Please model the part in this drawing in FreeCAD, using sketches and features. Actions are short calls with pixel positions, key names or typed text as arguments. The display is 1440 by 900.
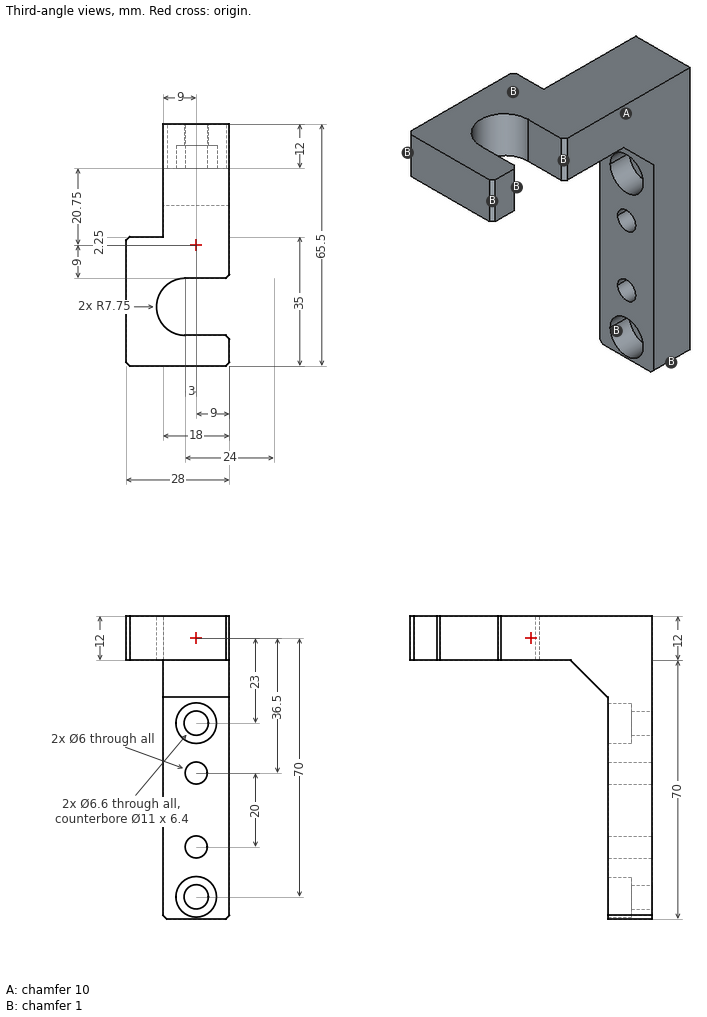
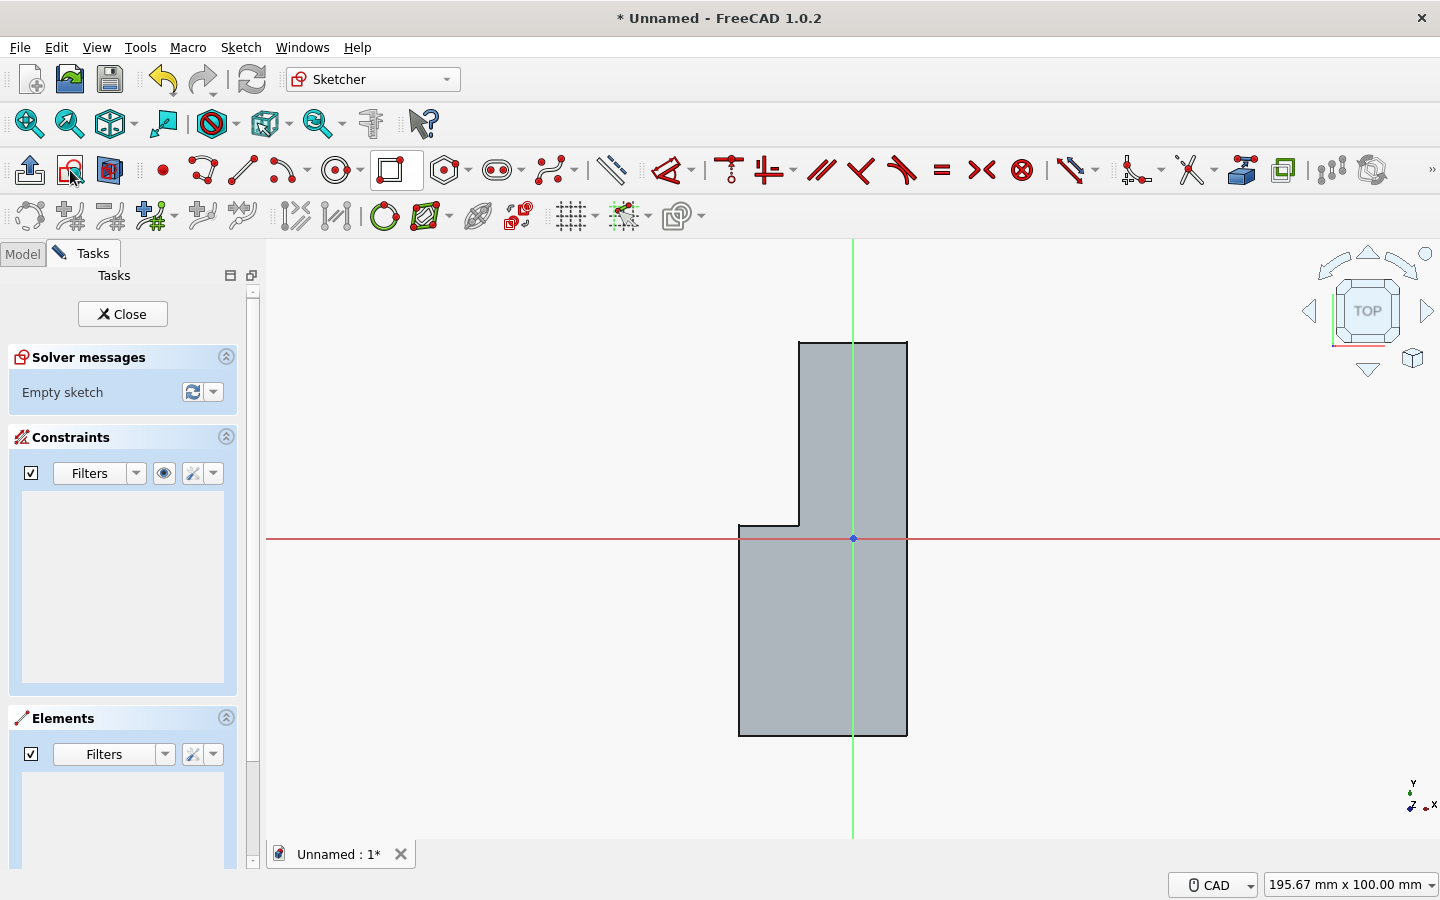
scroll(978, 655, up, 5)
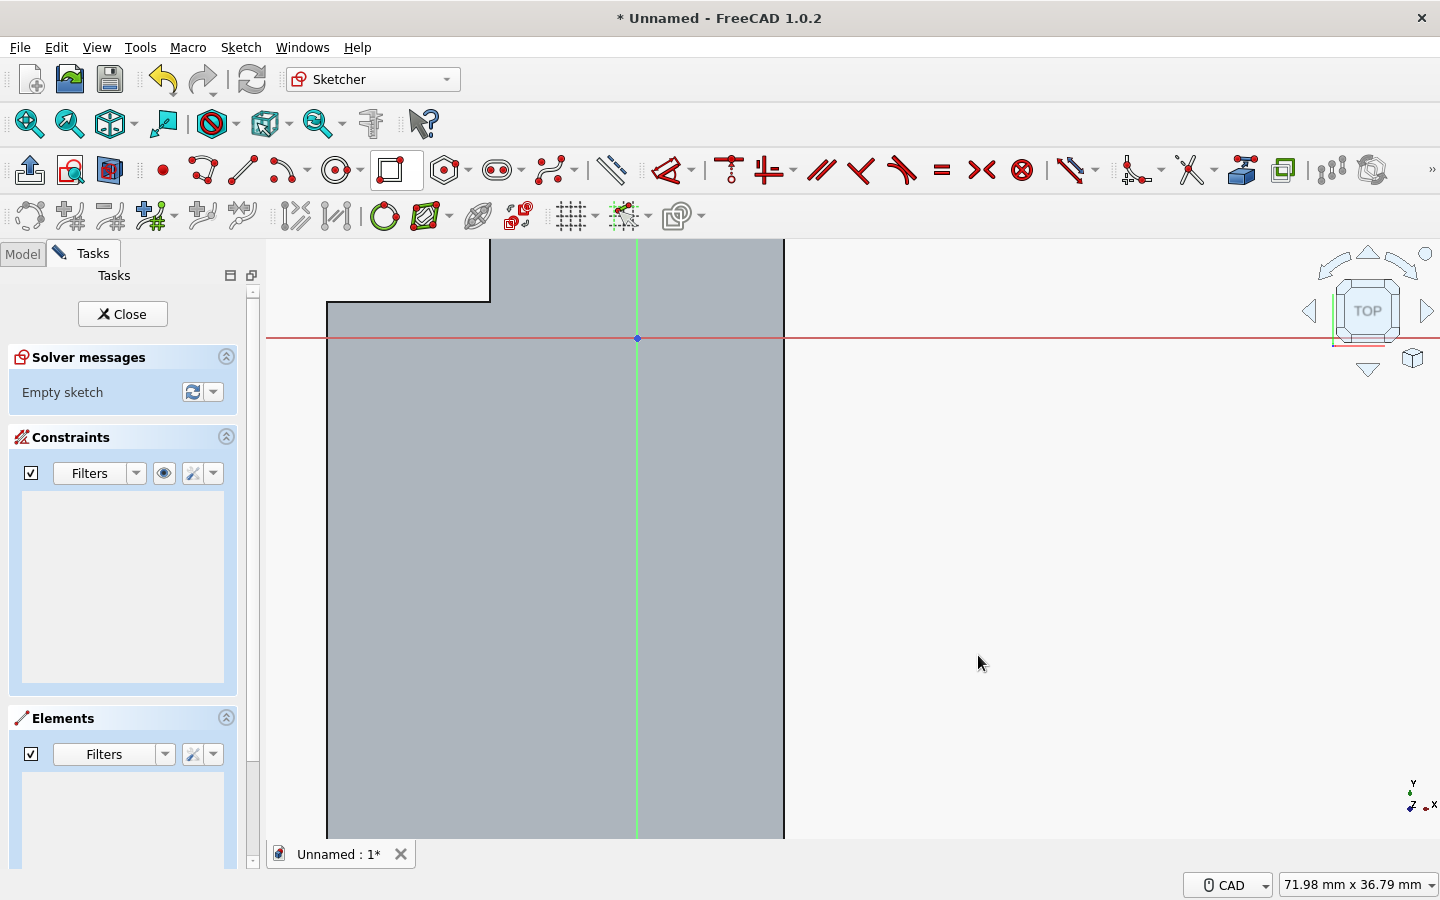
click(498, 170)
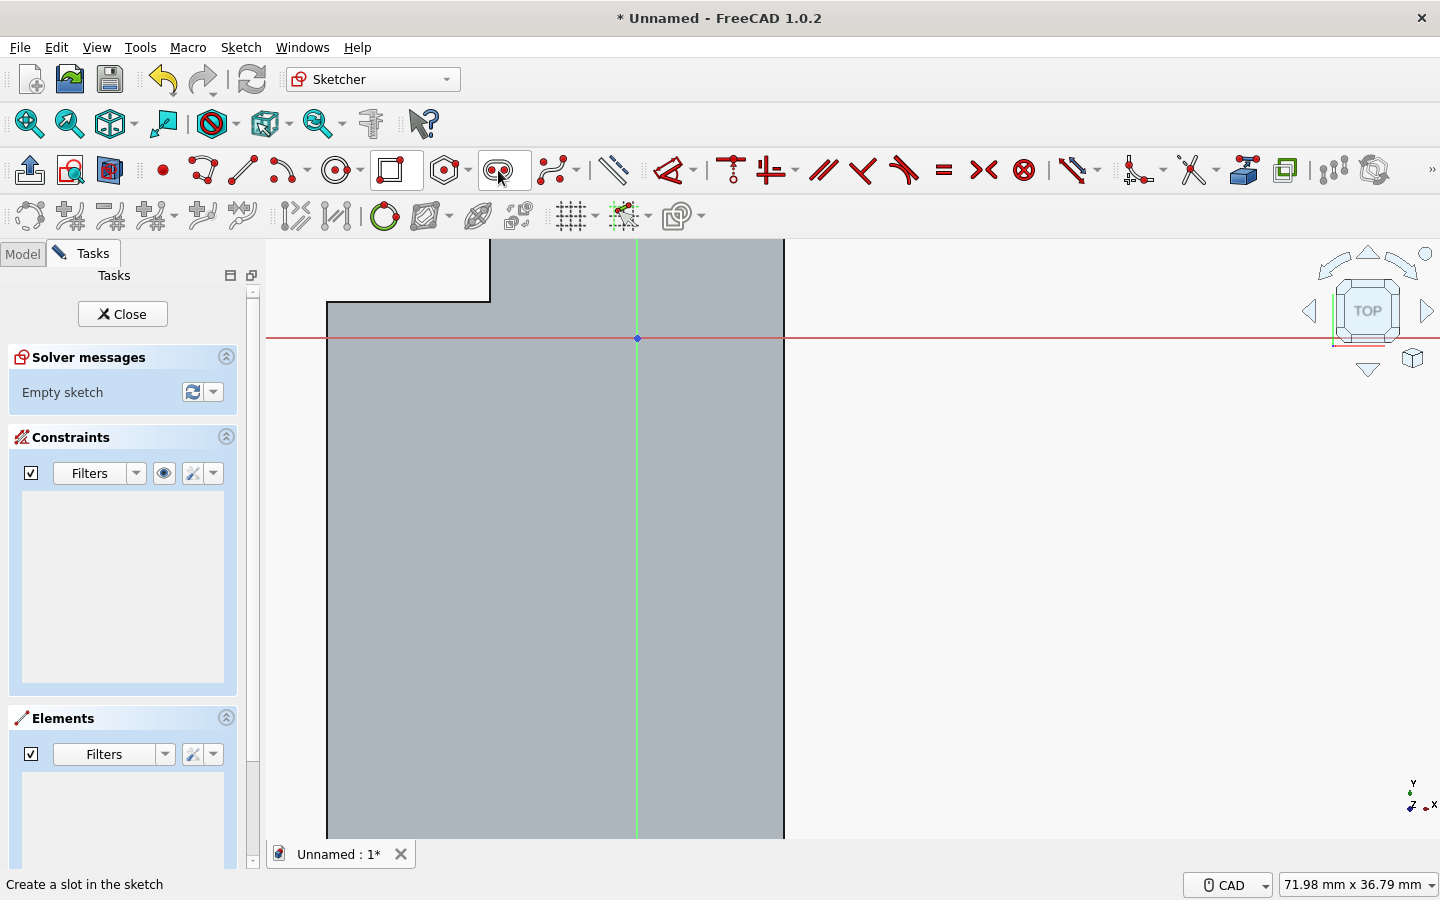
click(588, 612)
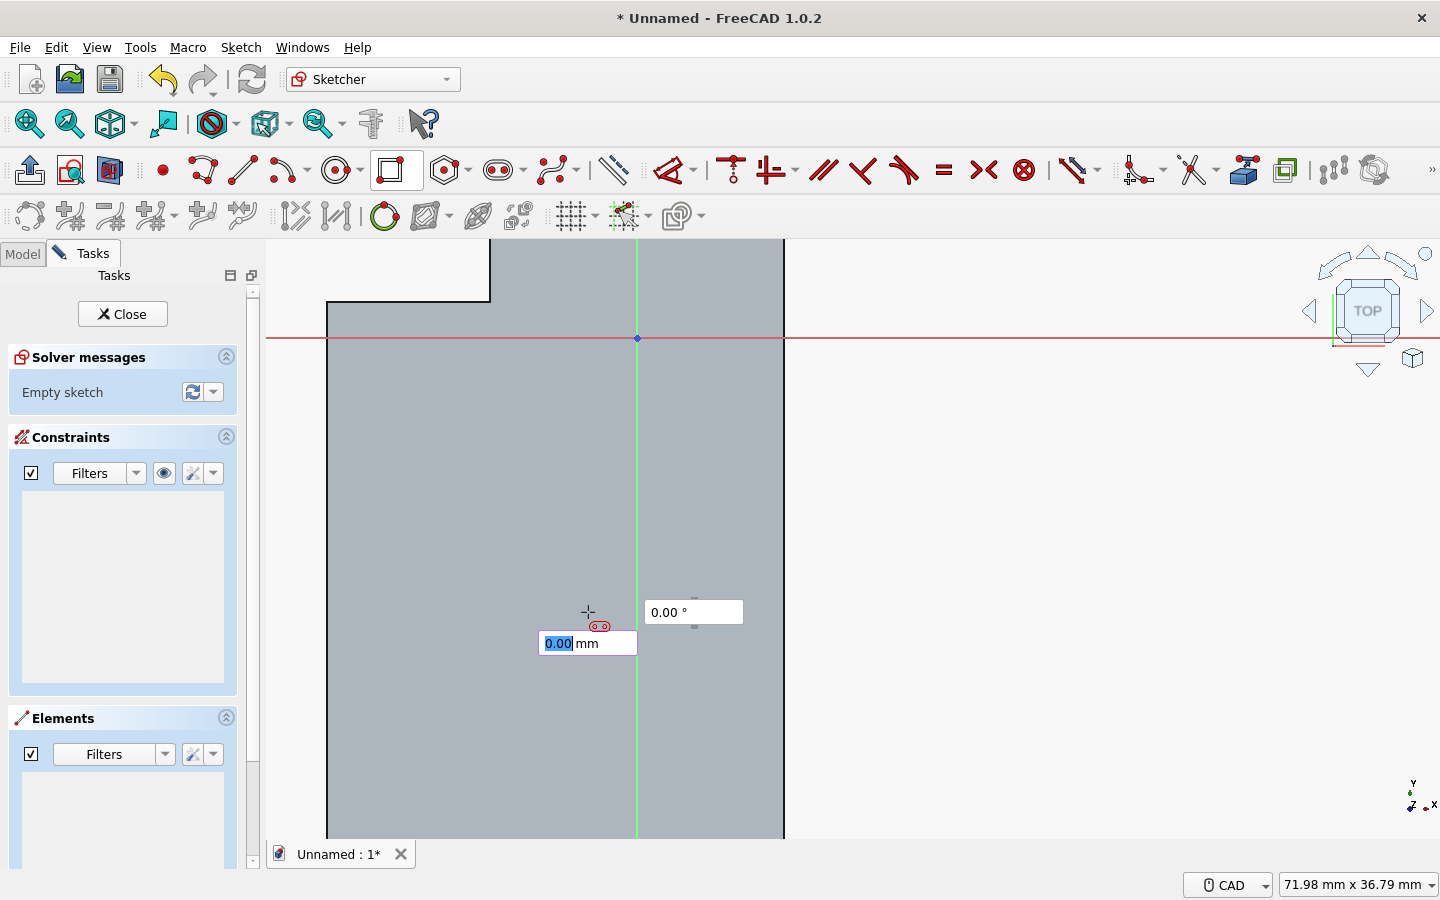
click(980, 612)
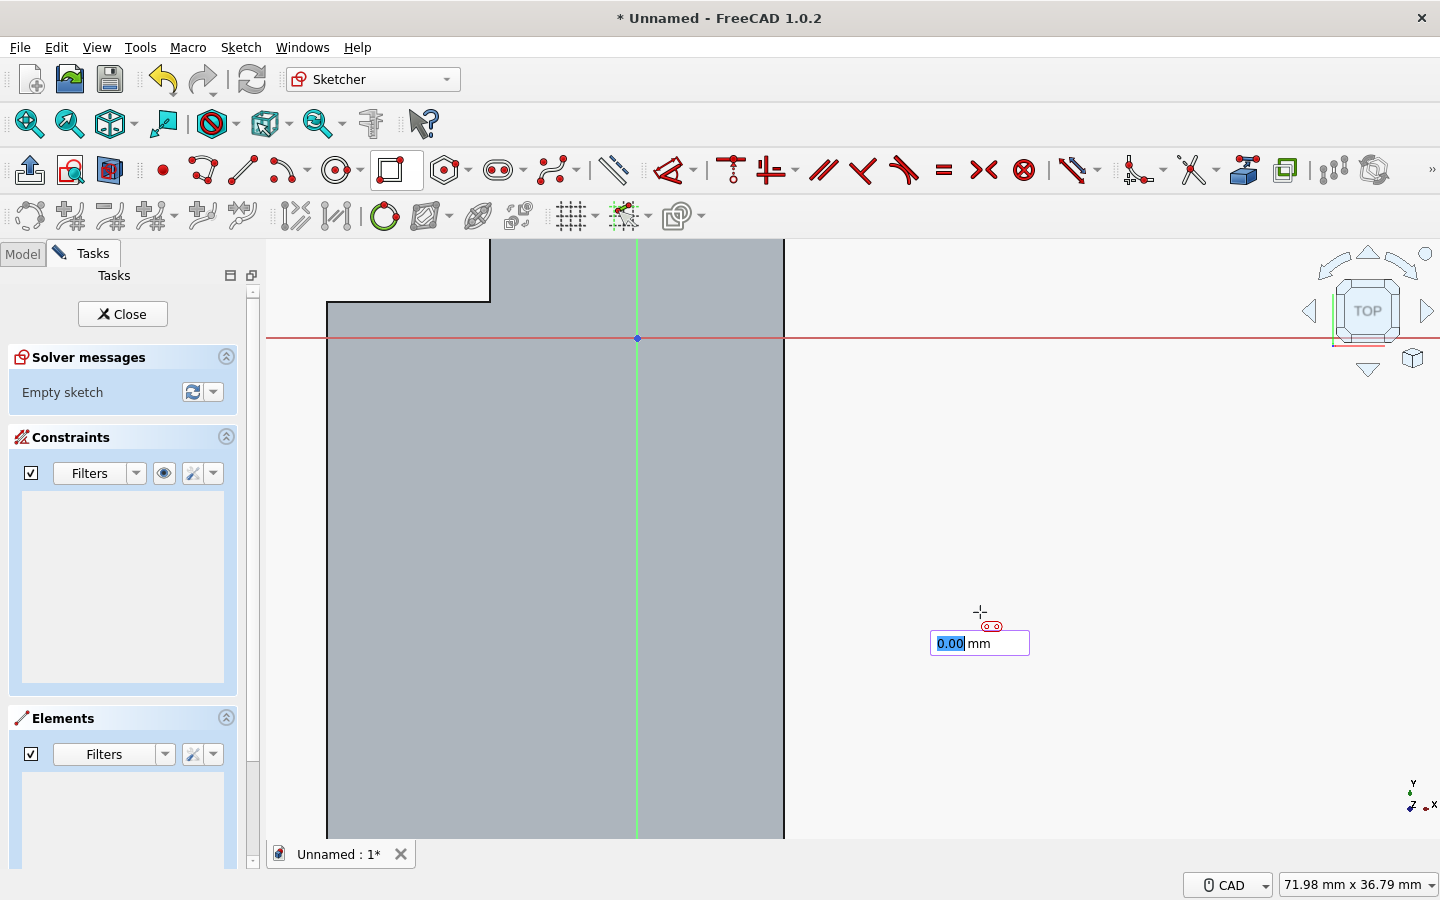
click(784, 485)
key(Escape)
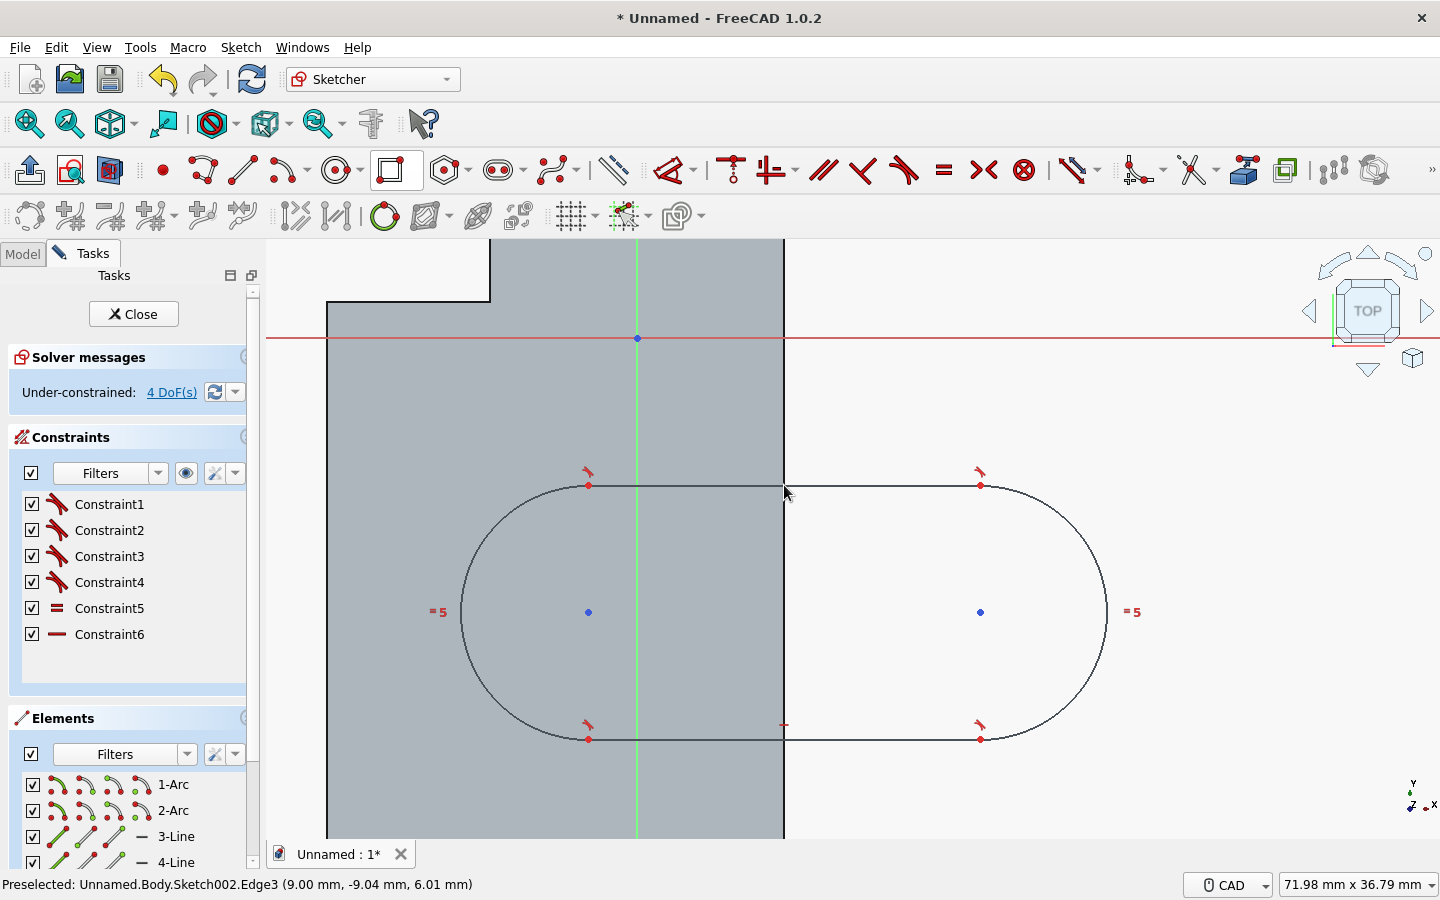
click(668, 170)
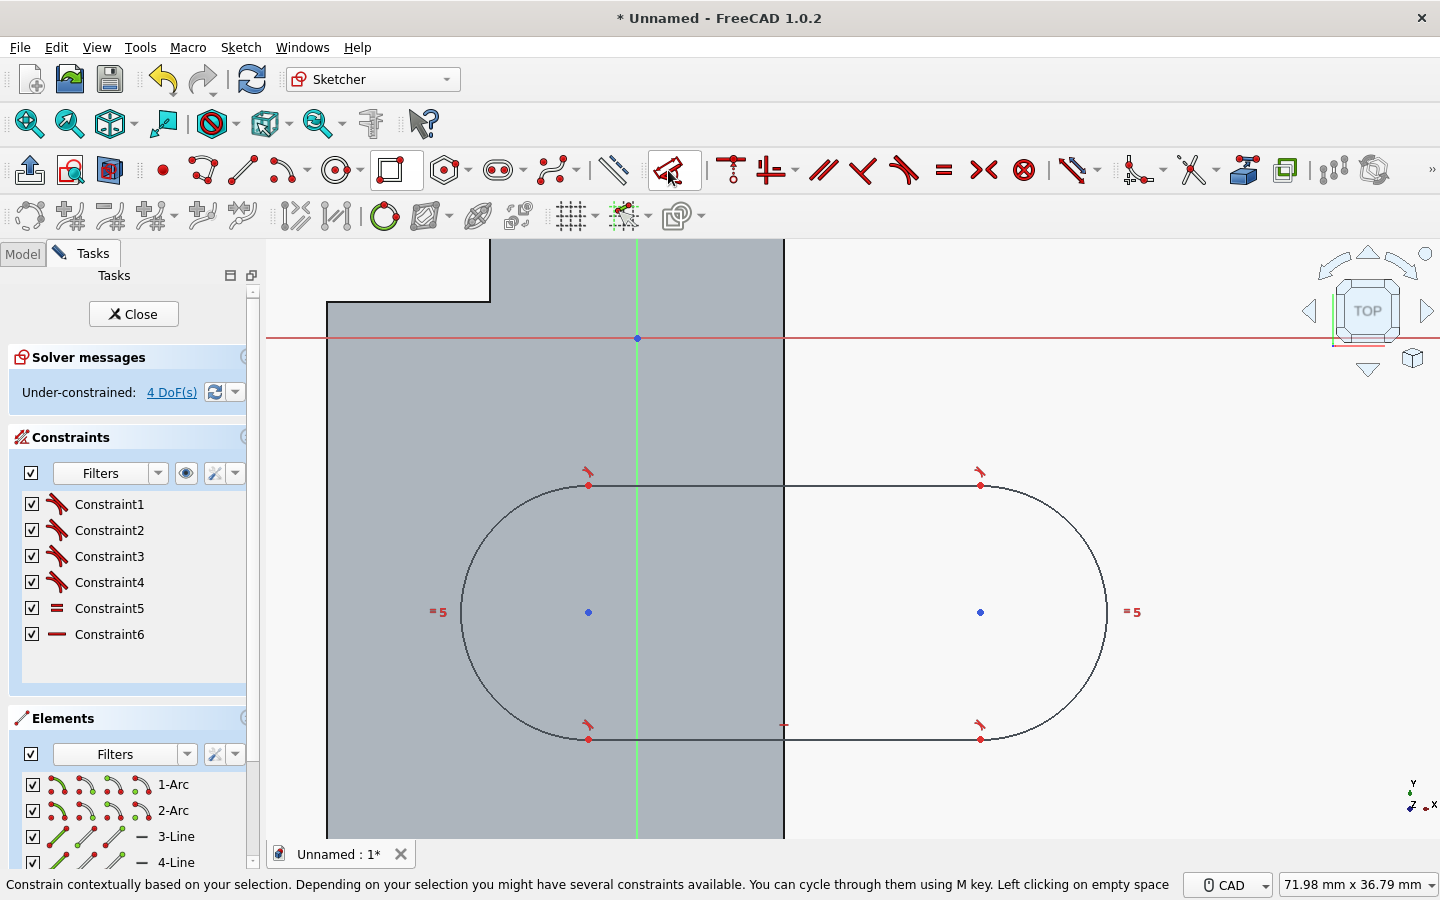
click(485, 538)
click(459, 519)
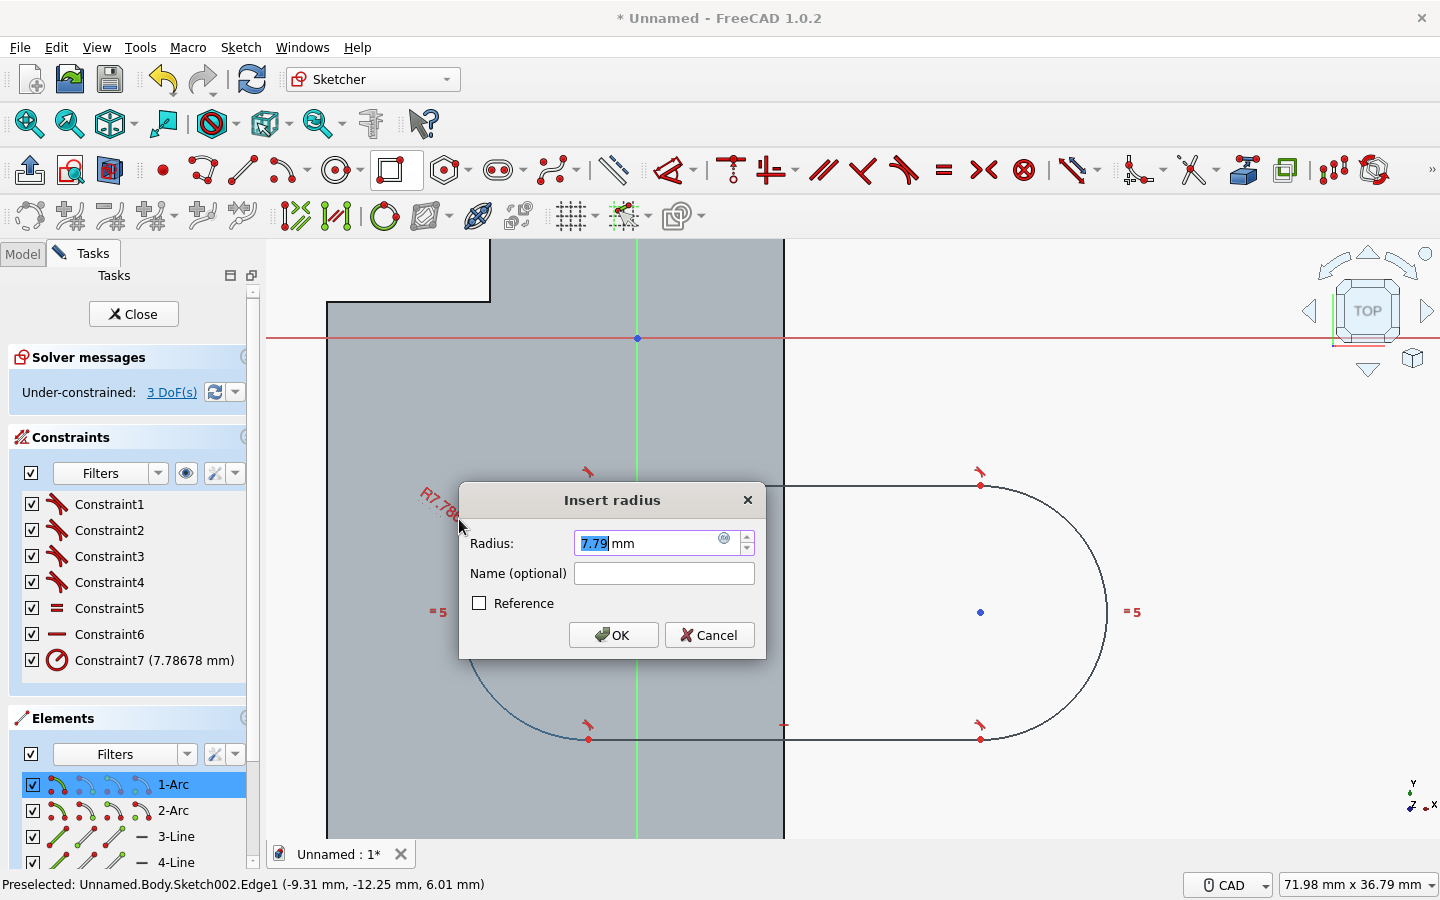
text(7.75)
key(Return)